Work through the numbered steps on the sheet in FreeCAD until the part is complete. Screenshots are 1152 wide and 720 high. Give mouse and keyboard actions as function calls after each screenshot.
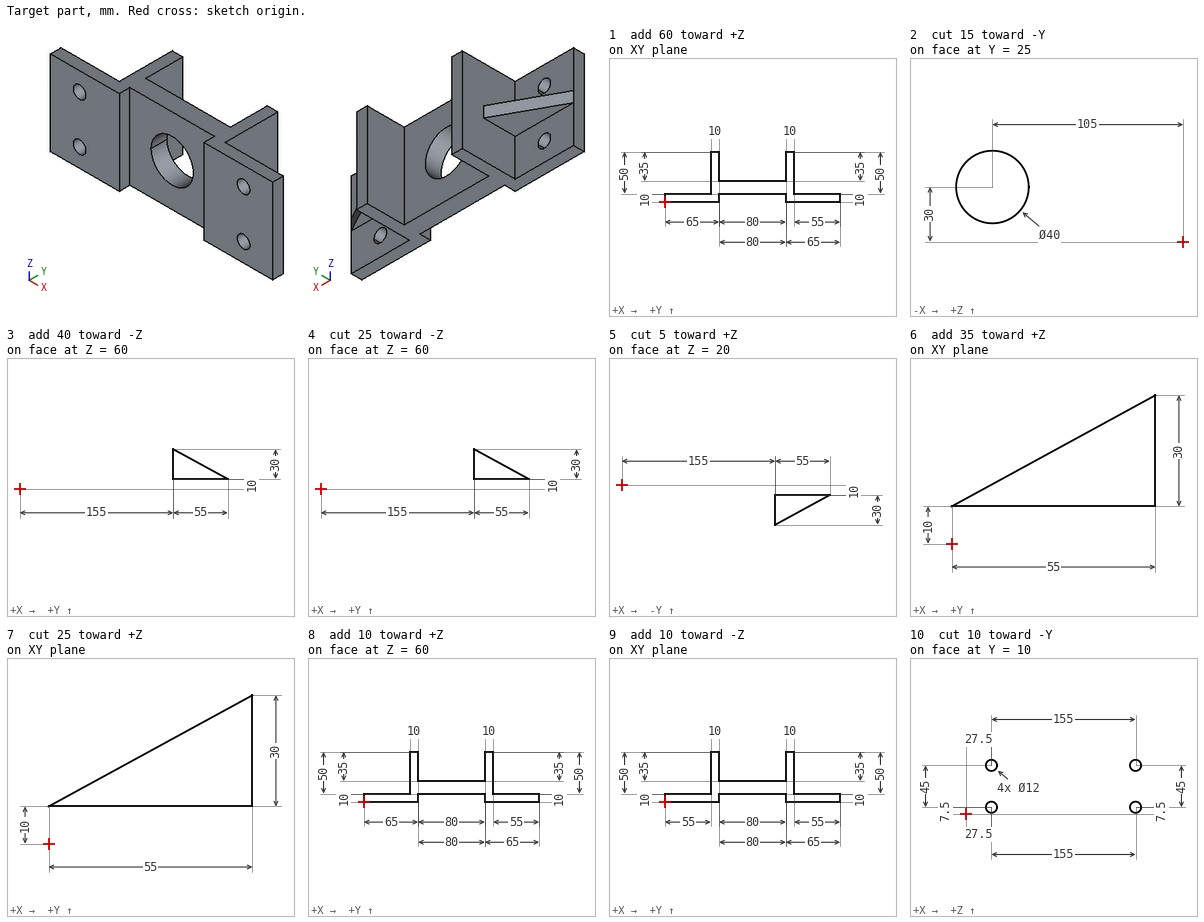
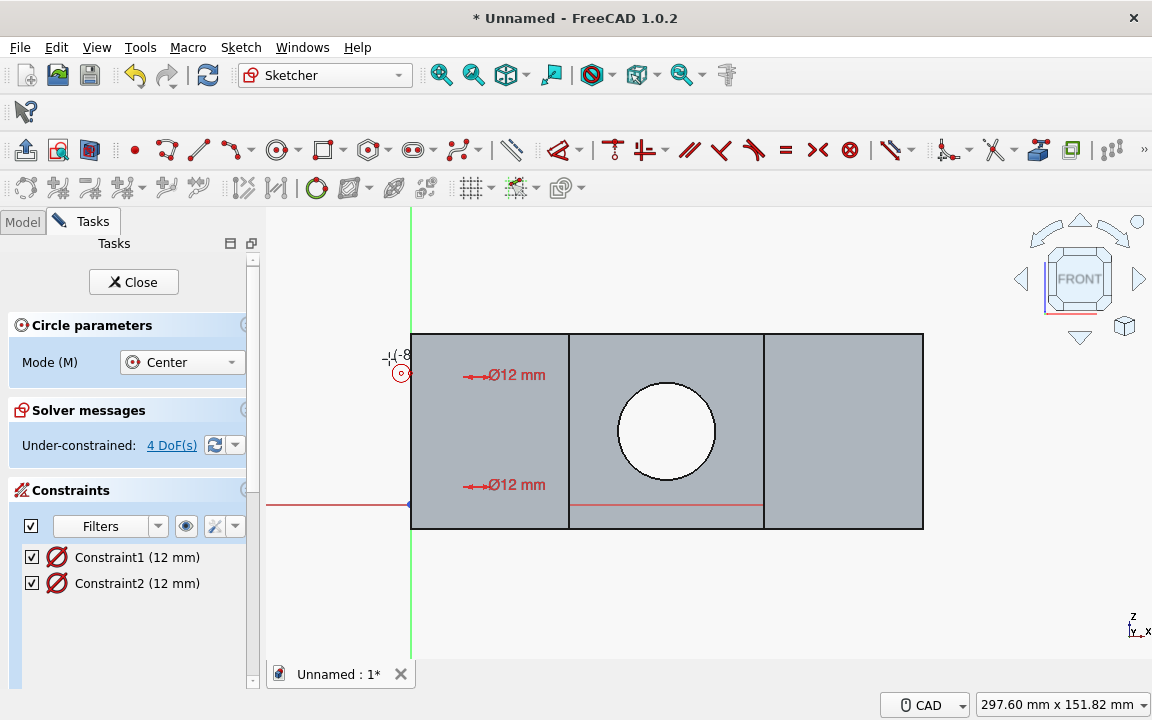
scroll(856, 486, up, 3)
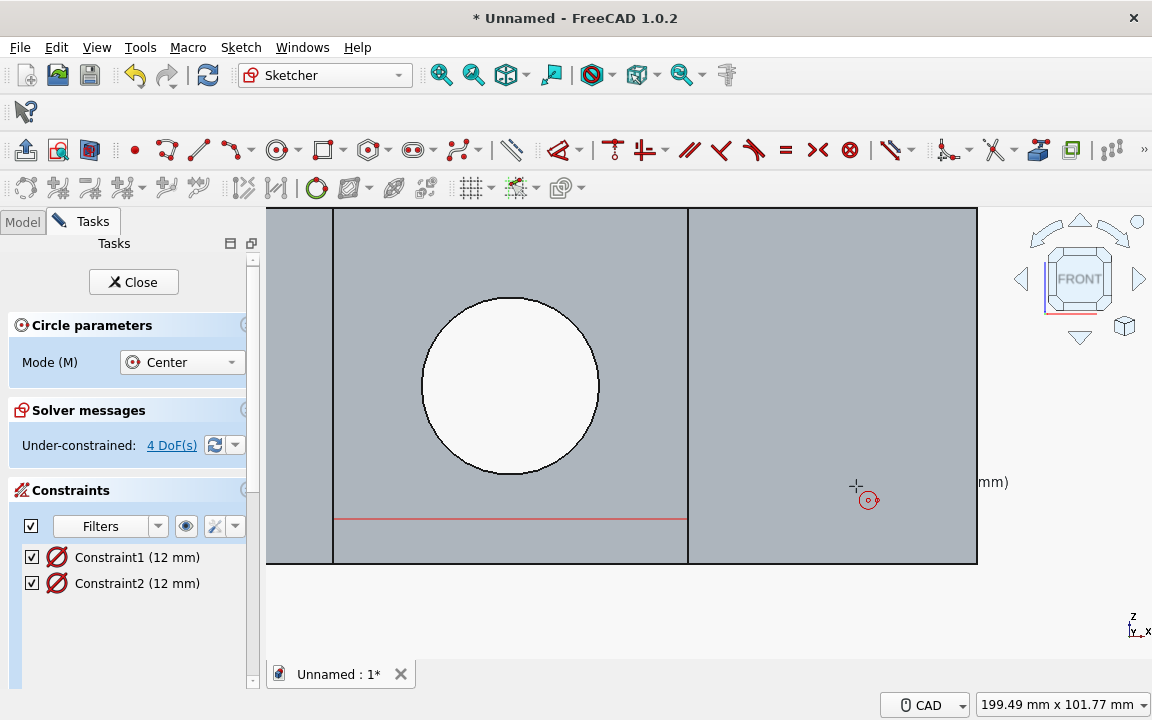
click(855, 486)
move(873, 467)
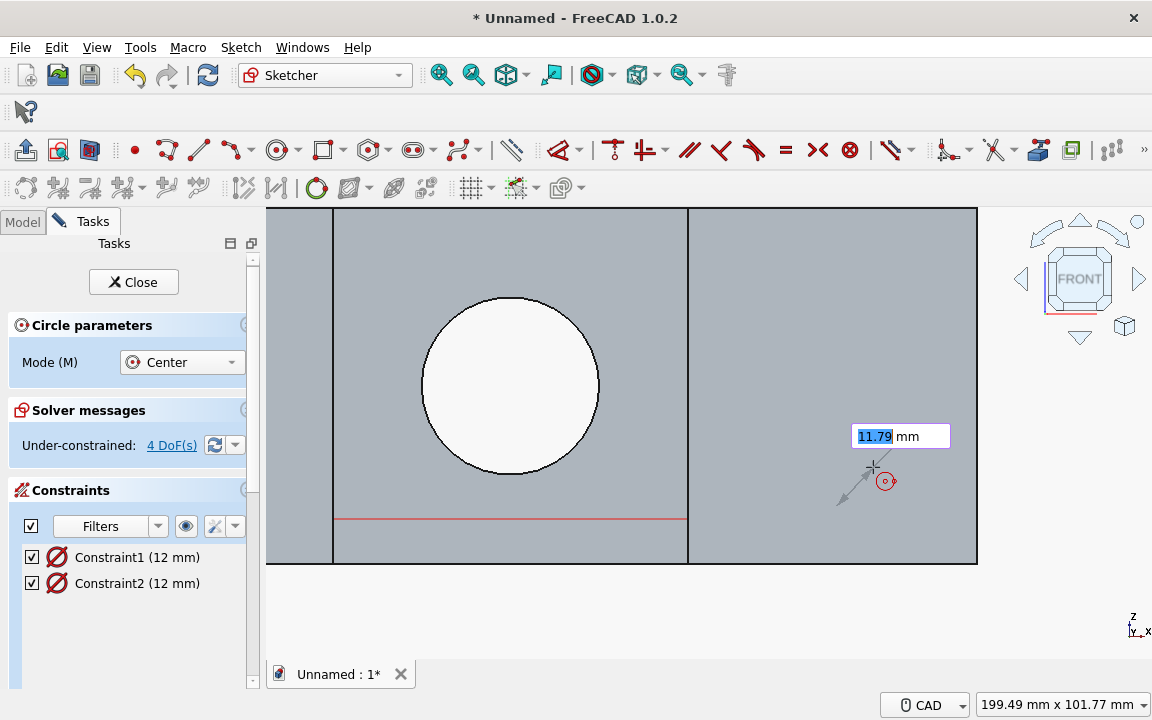
text(12)
key(Return)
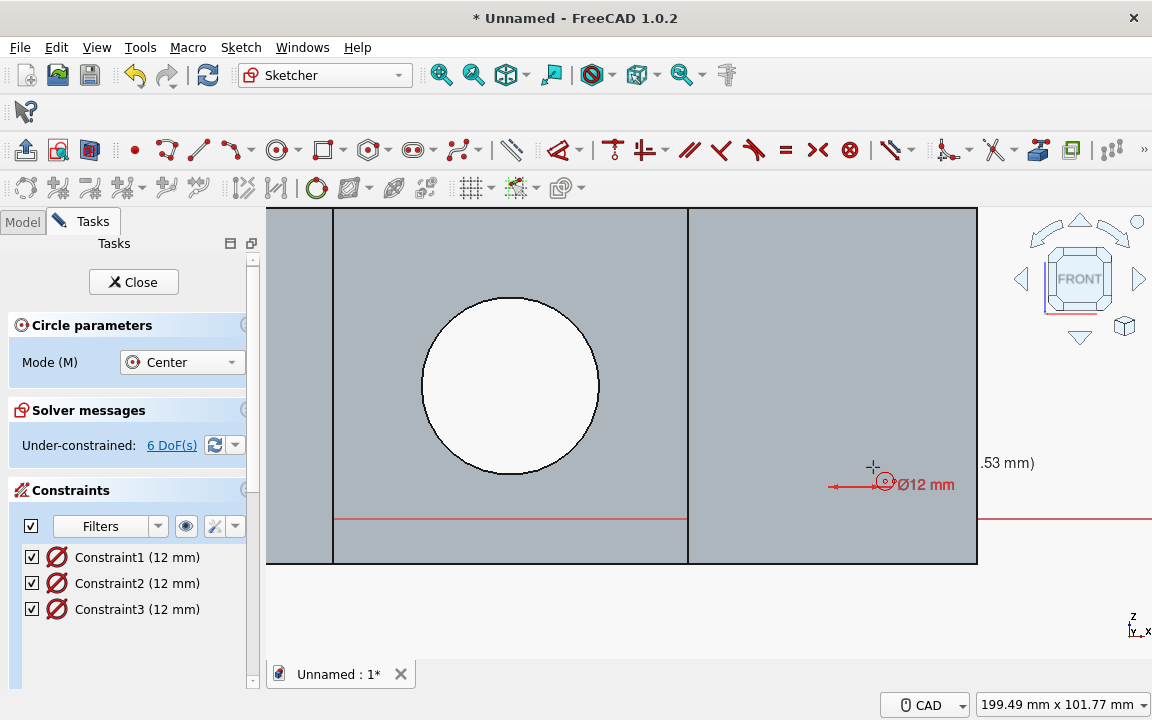
click(855, 286)
move(873, 267)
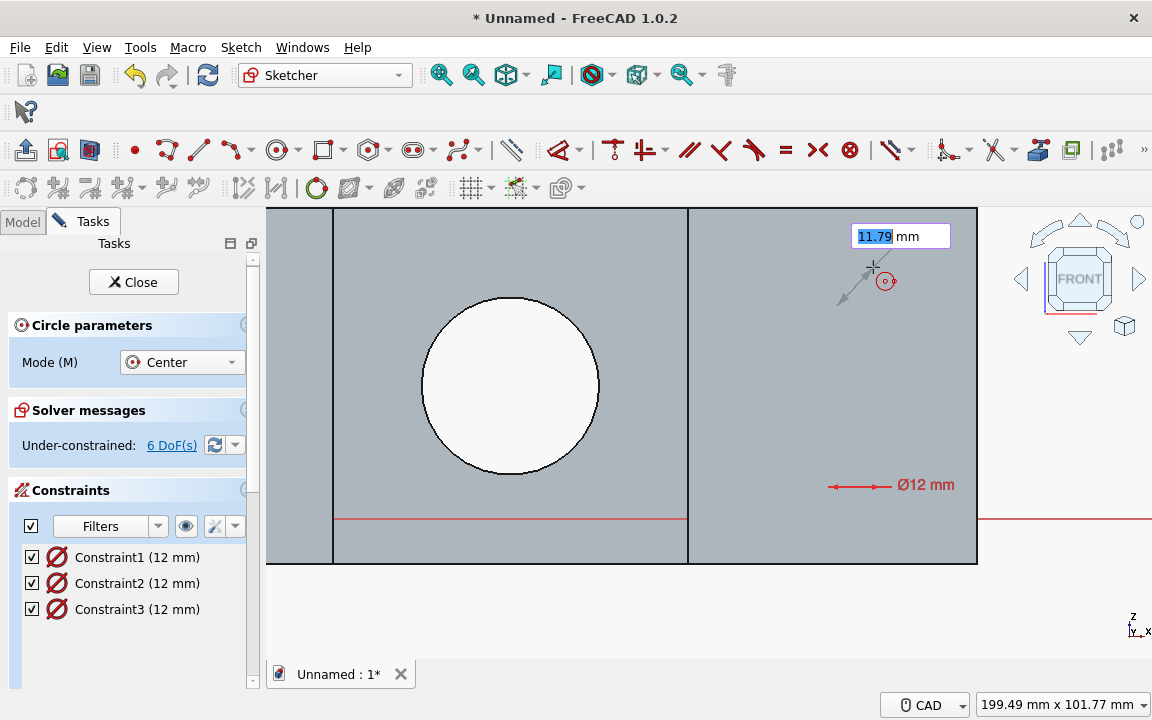
text(12)
key(Return)
key(Escape)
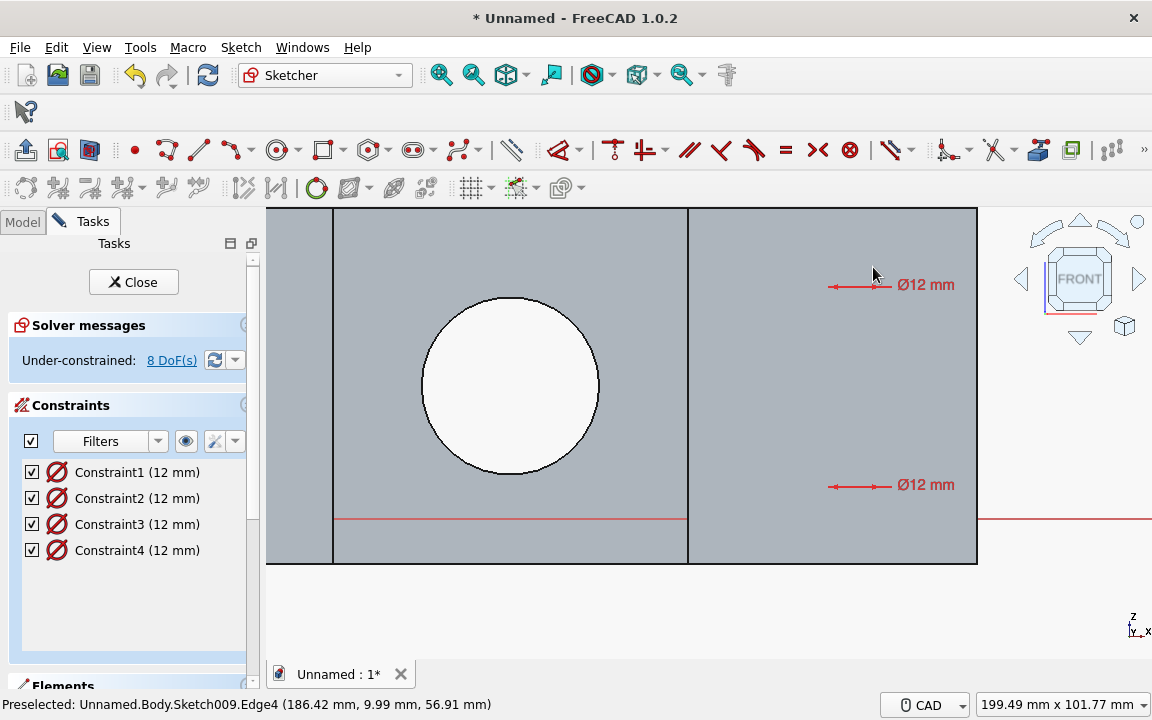
key(d)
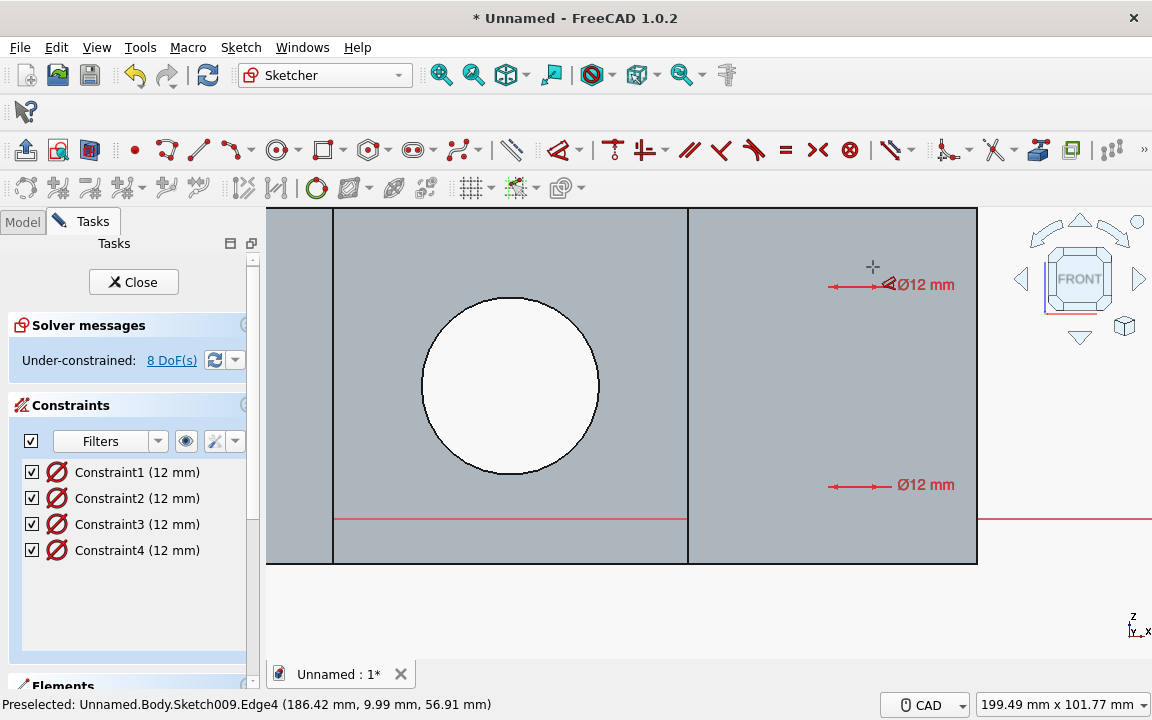
scroll(857, 486, down, 3)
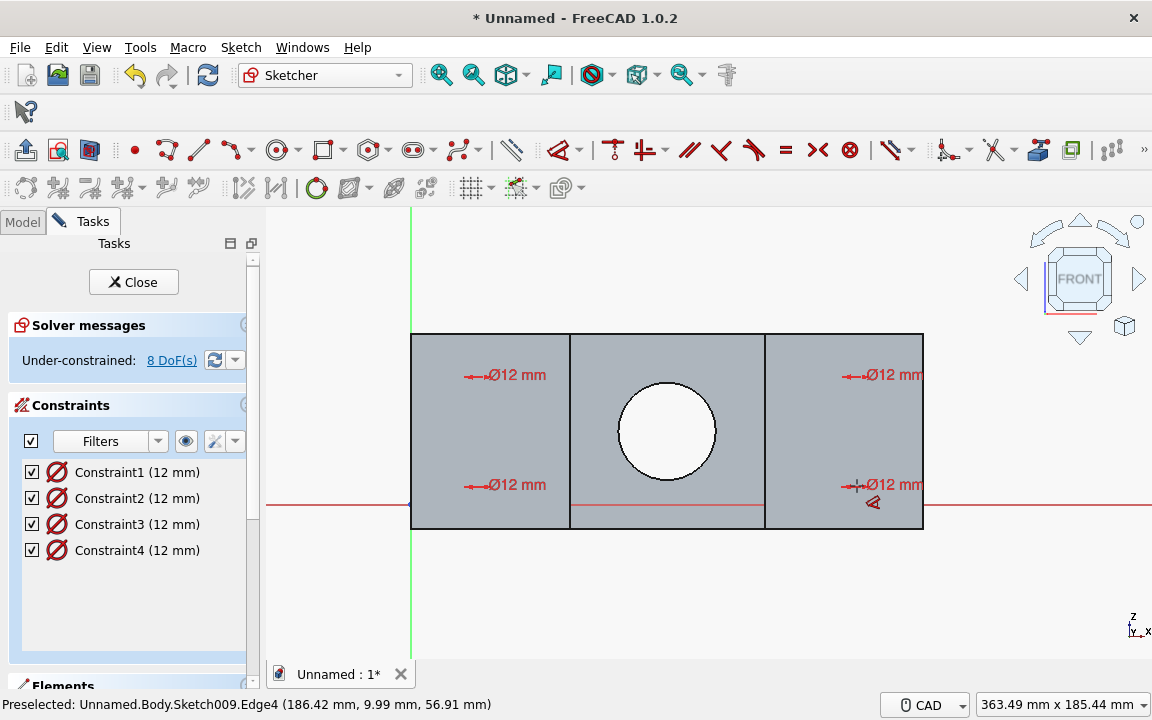
scroll(478, 487, up, 4)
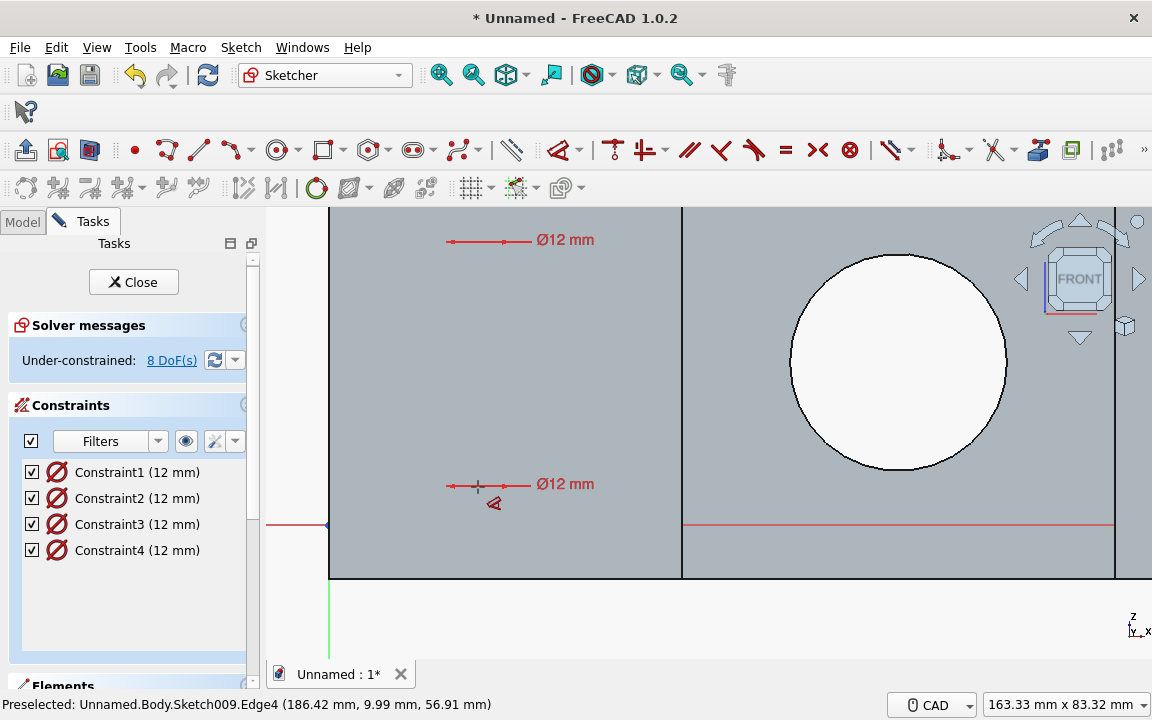
click(479, 486)
click(295, 506)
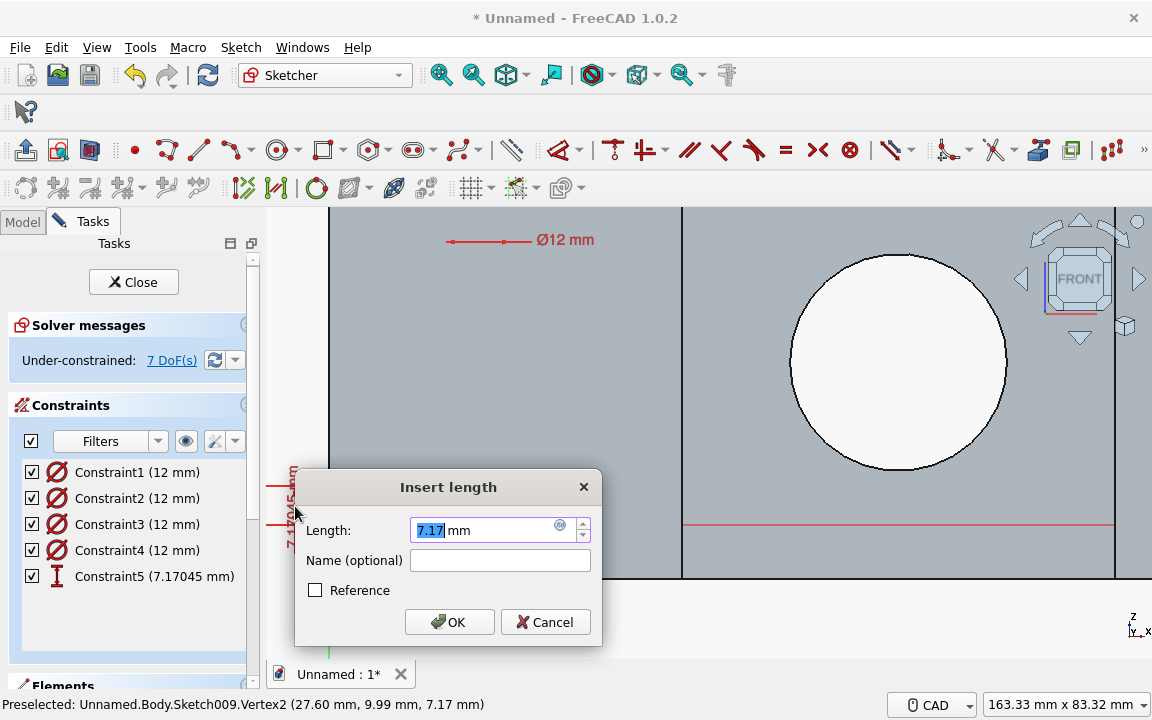
text(7.5)
key(Return)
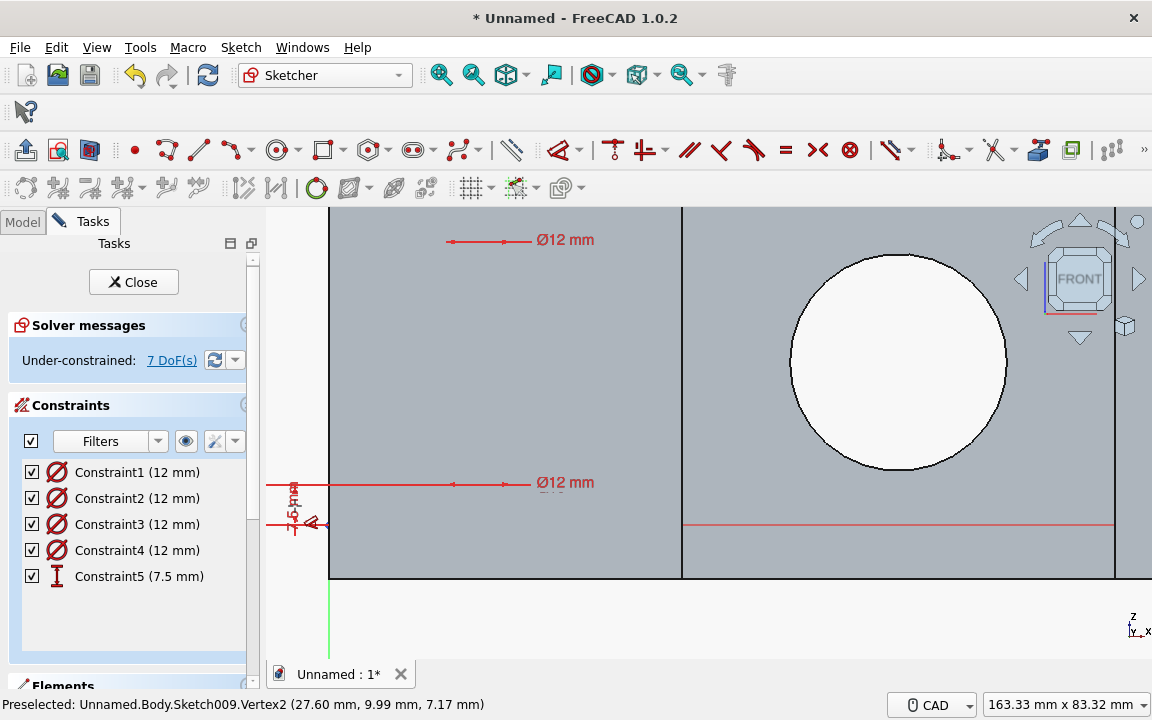
scroll(478, 487, down, 4)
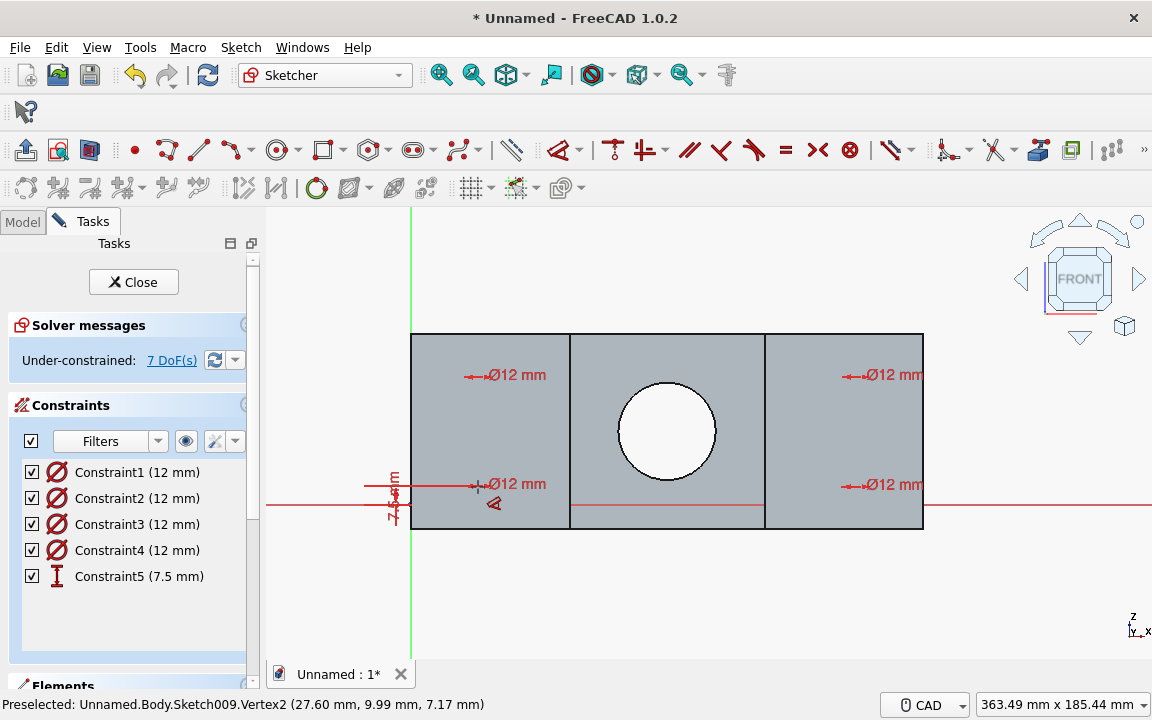
scroll(856, 487, up, 4)